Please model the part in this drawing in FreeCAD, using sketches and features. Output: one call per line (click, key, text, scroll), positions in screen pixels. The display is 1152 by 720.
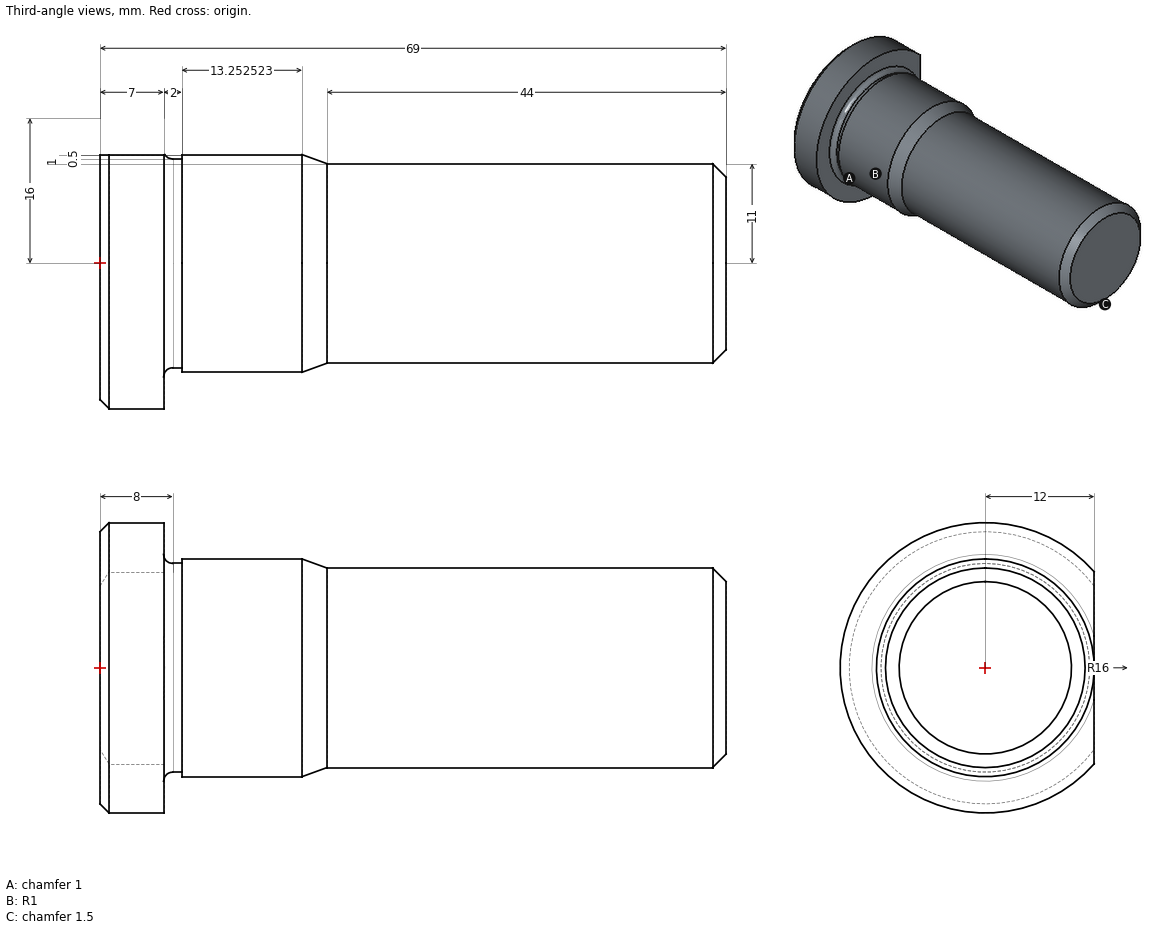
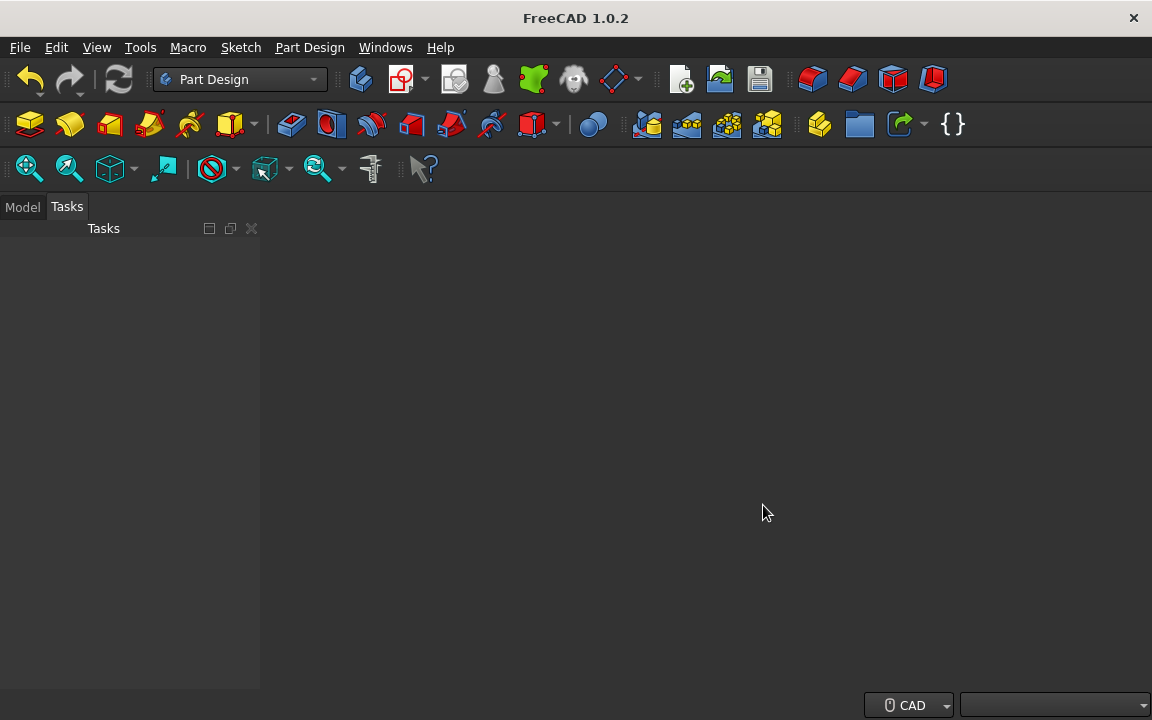
click(680, 80)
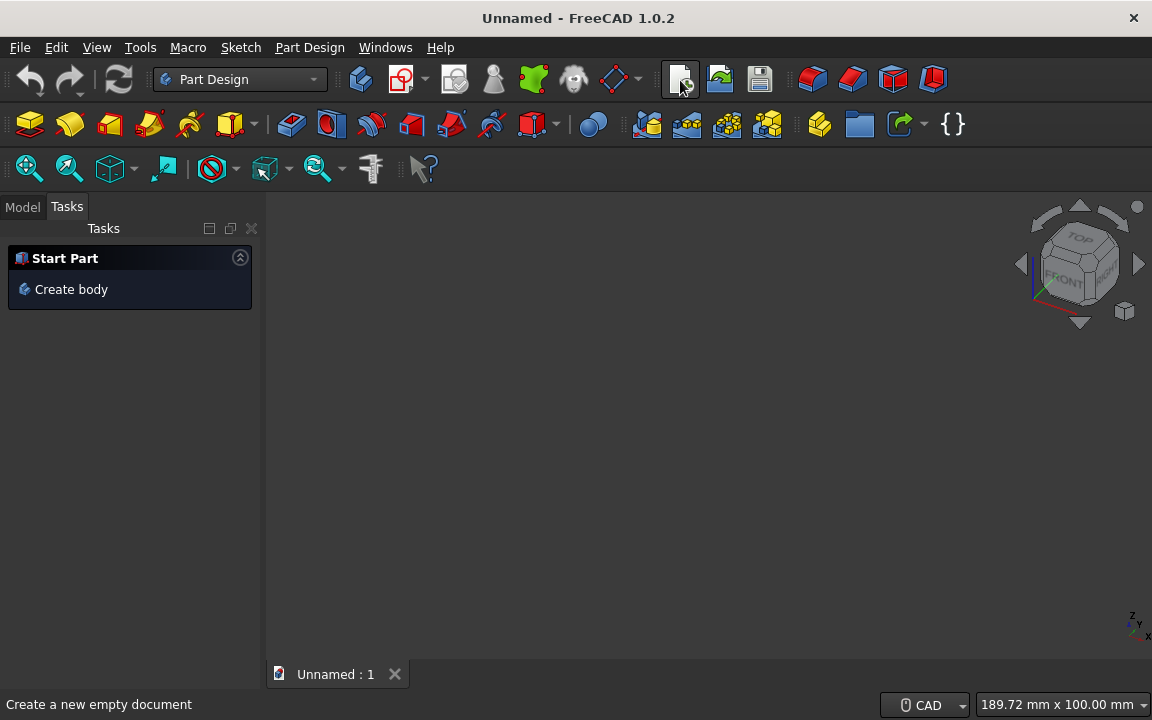
click(402, 80)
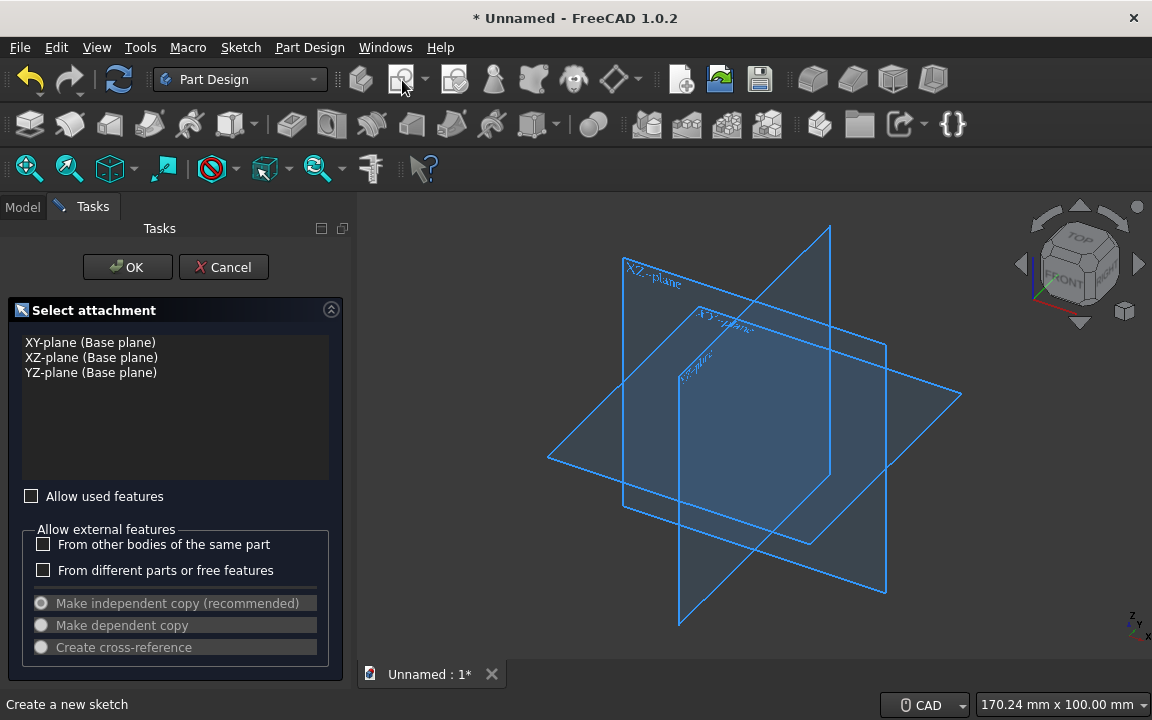
click(82, 342)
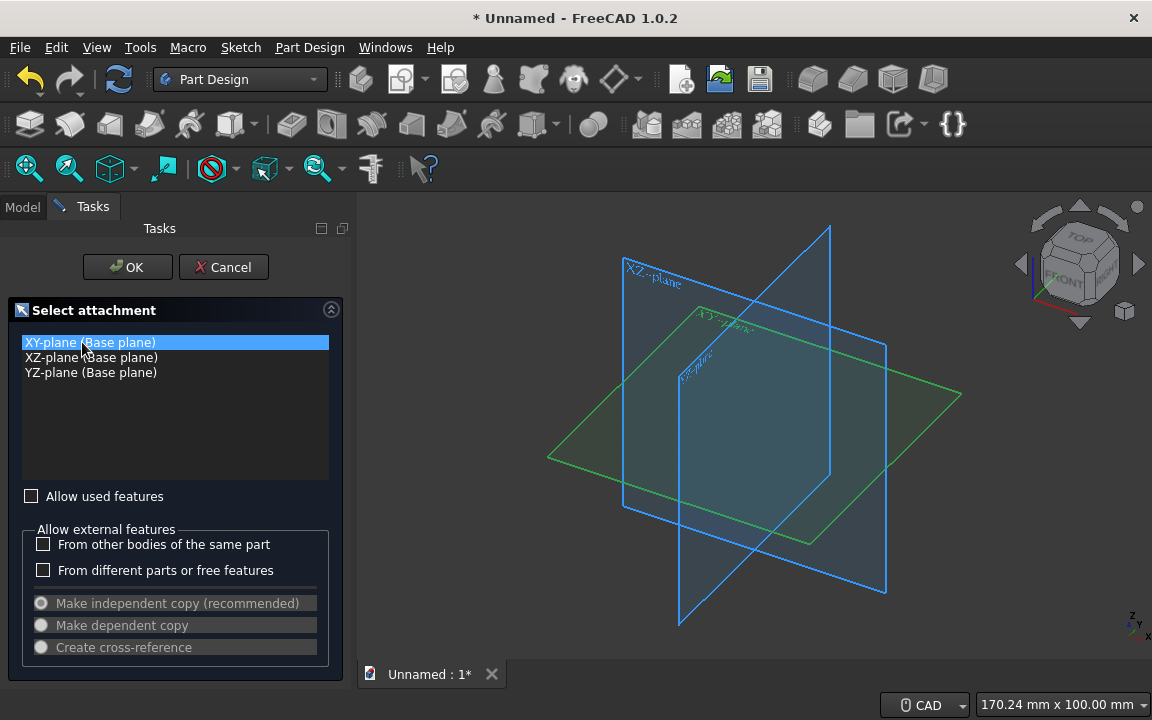
click(128, 267)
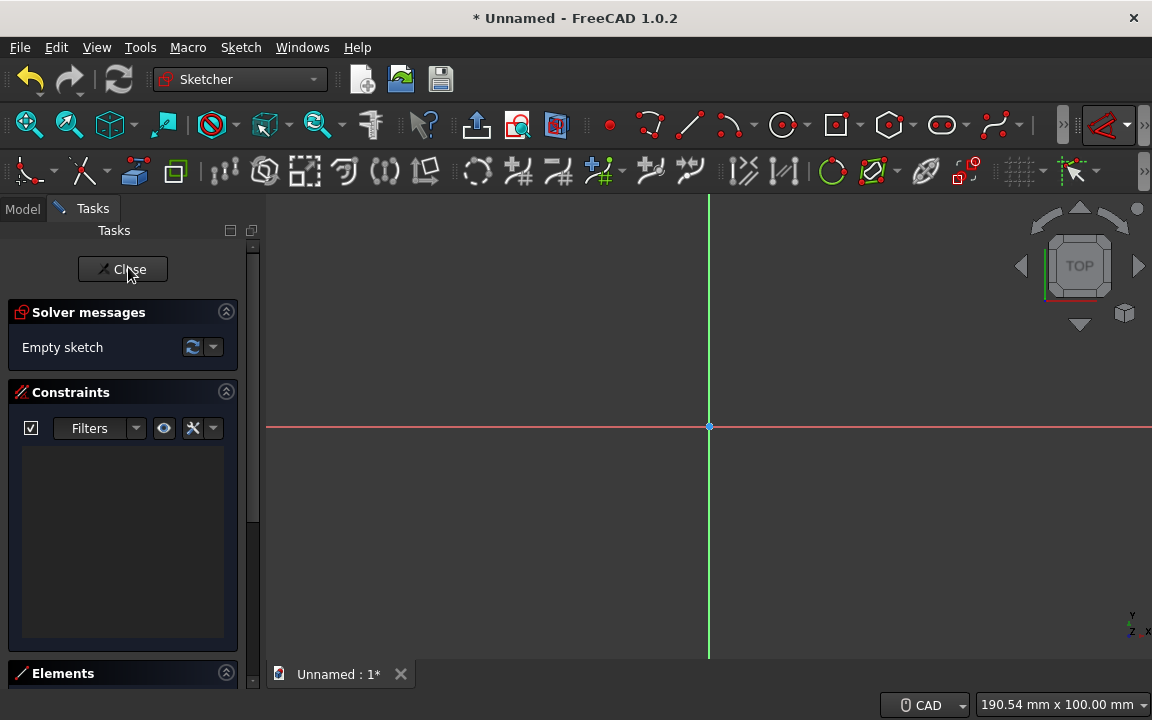
scroll(294, 595, down, 1)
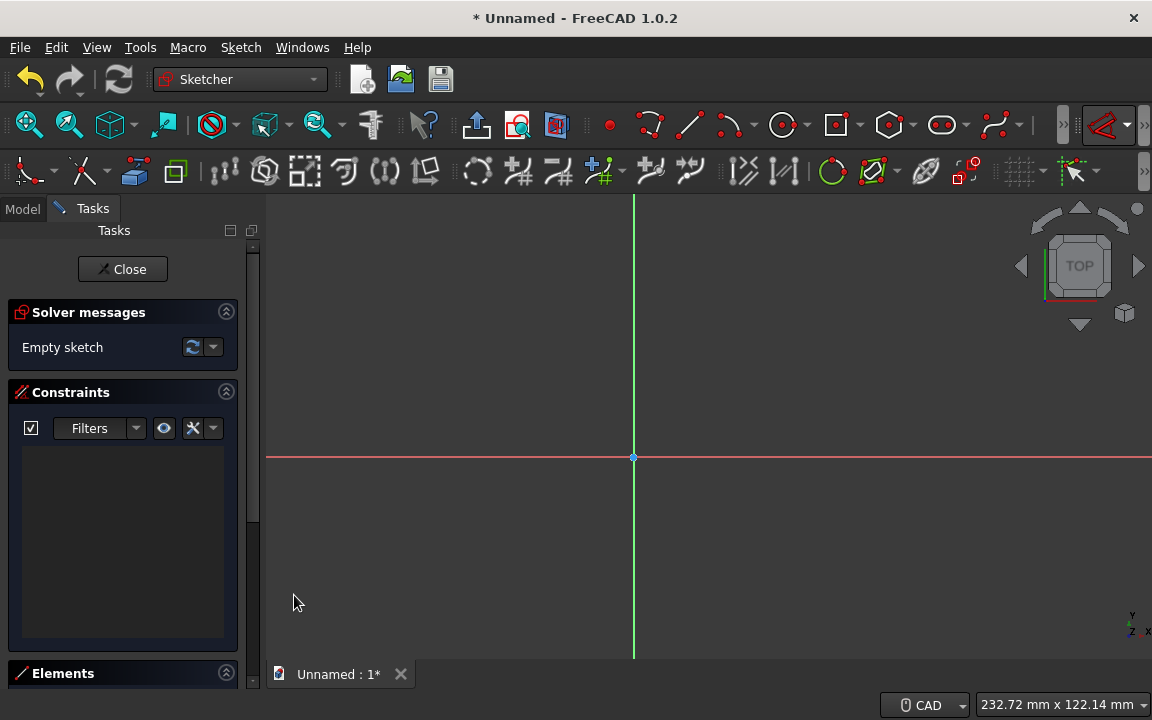
scroll(917, 427, up, 3)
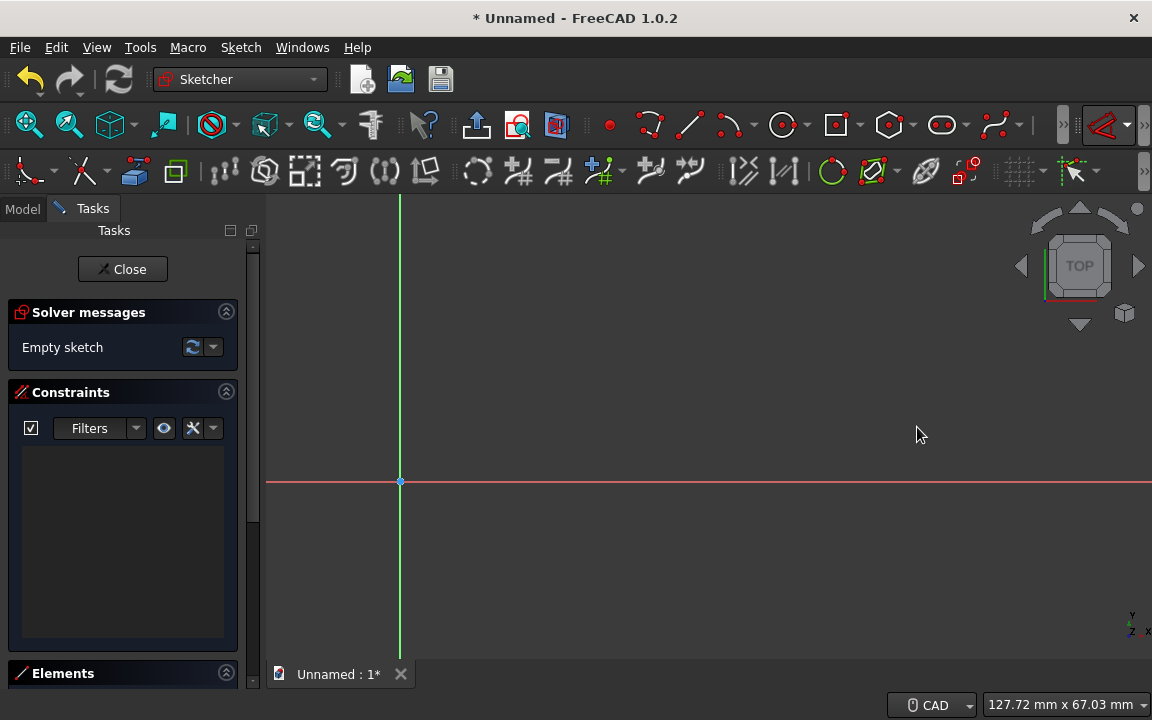
click(650, 126)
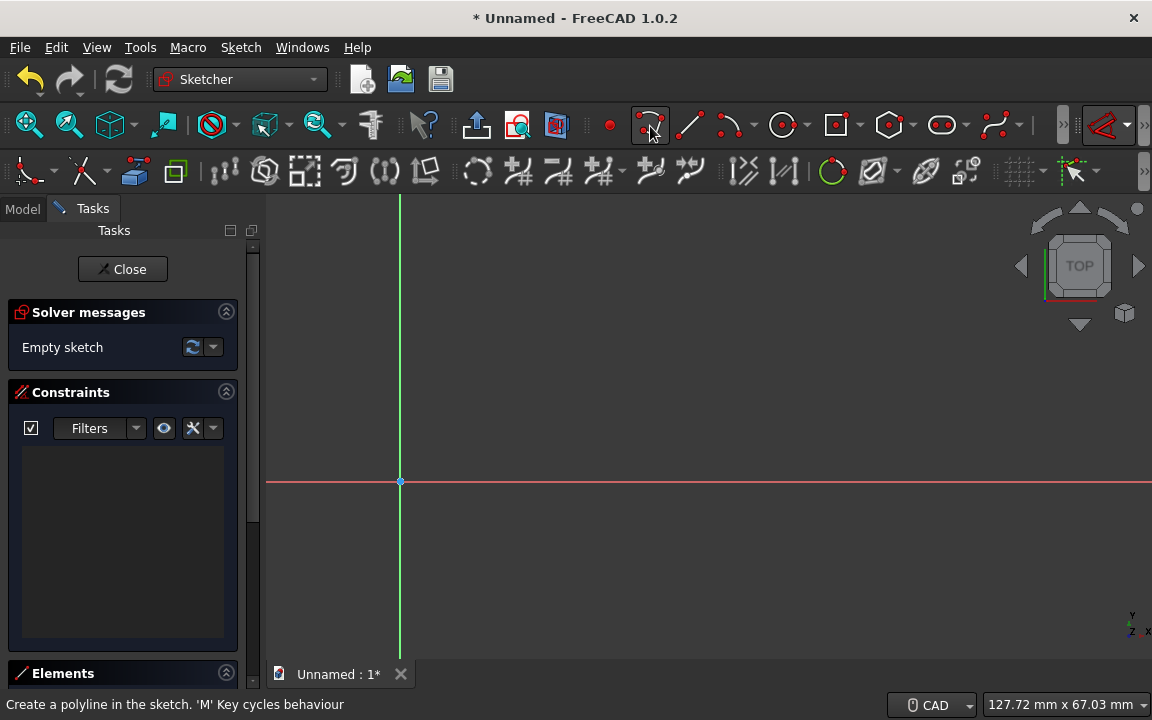
click(400, 482)
click(879, 473)
click(879, 405)
click(574, 405)
click(555, 398)
click(463, 398)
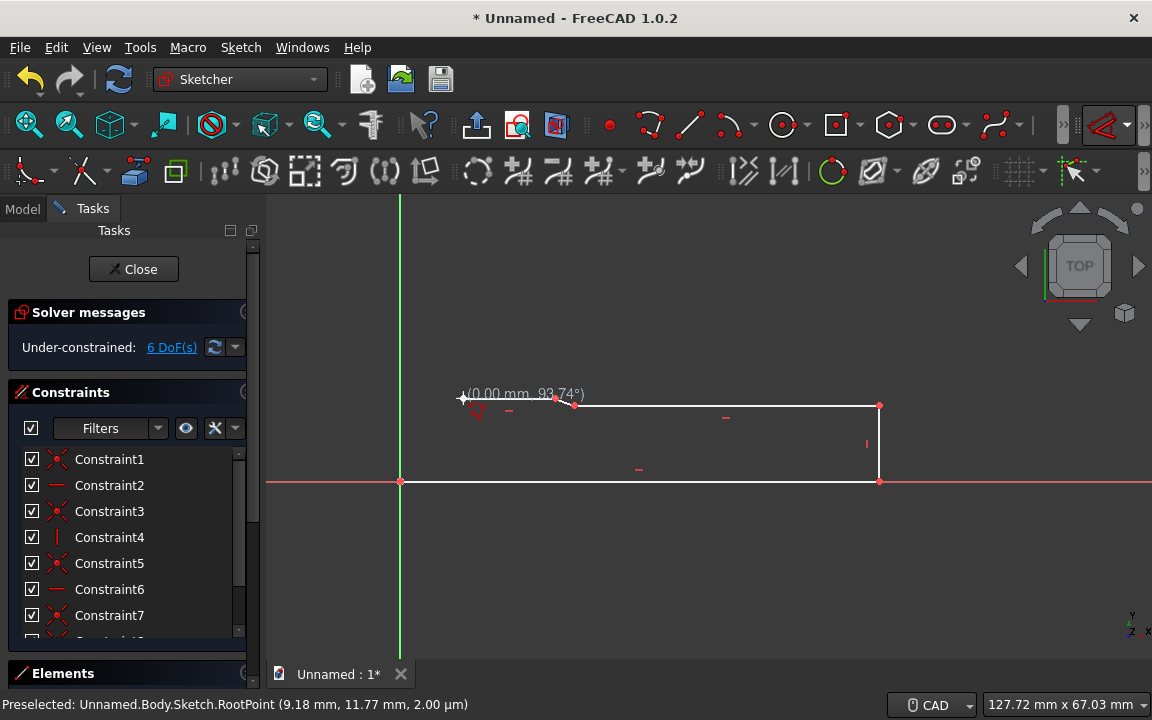
scroll(463, 402, up, 8)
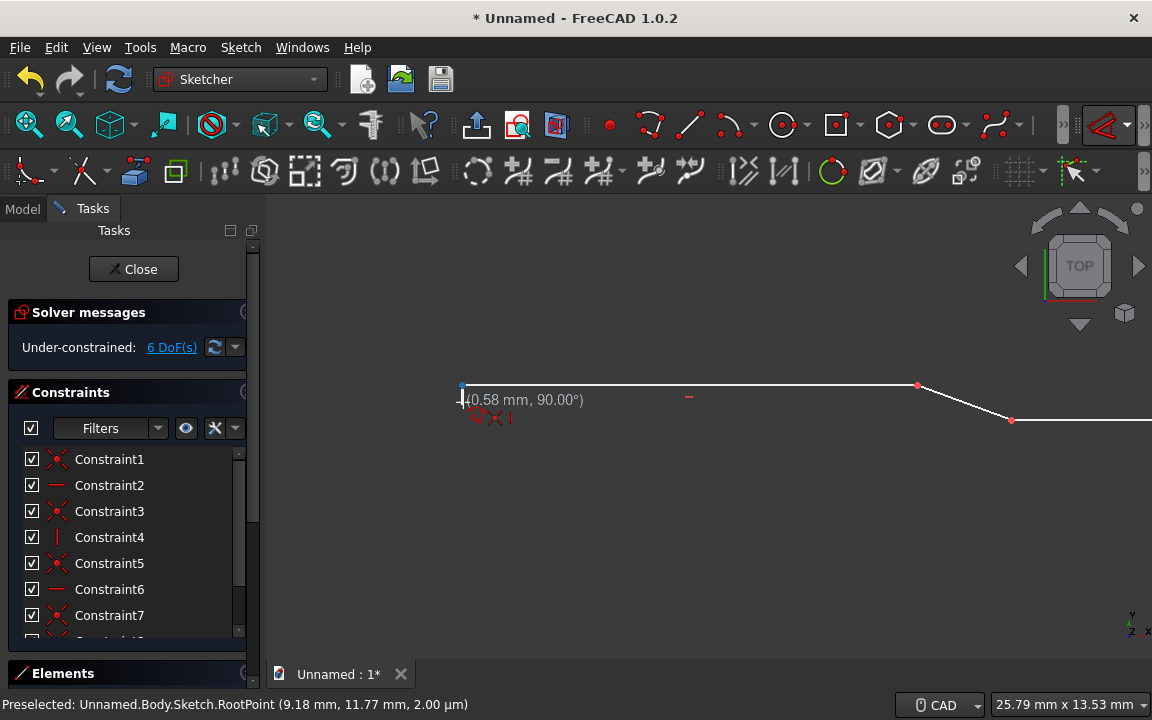
click(462, 399)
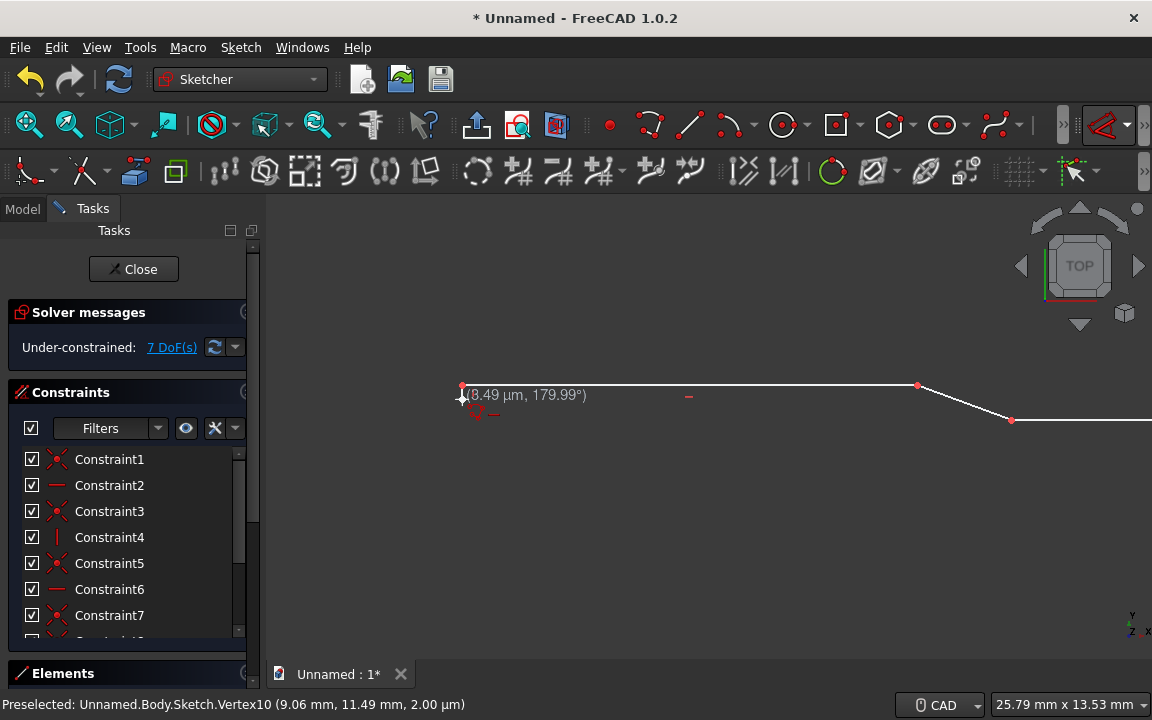
scroll(464, 403, down, 8)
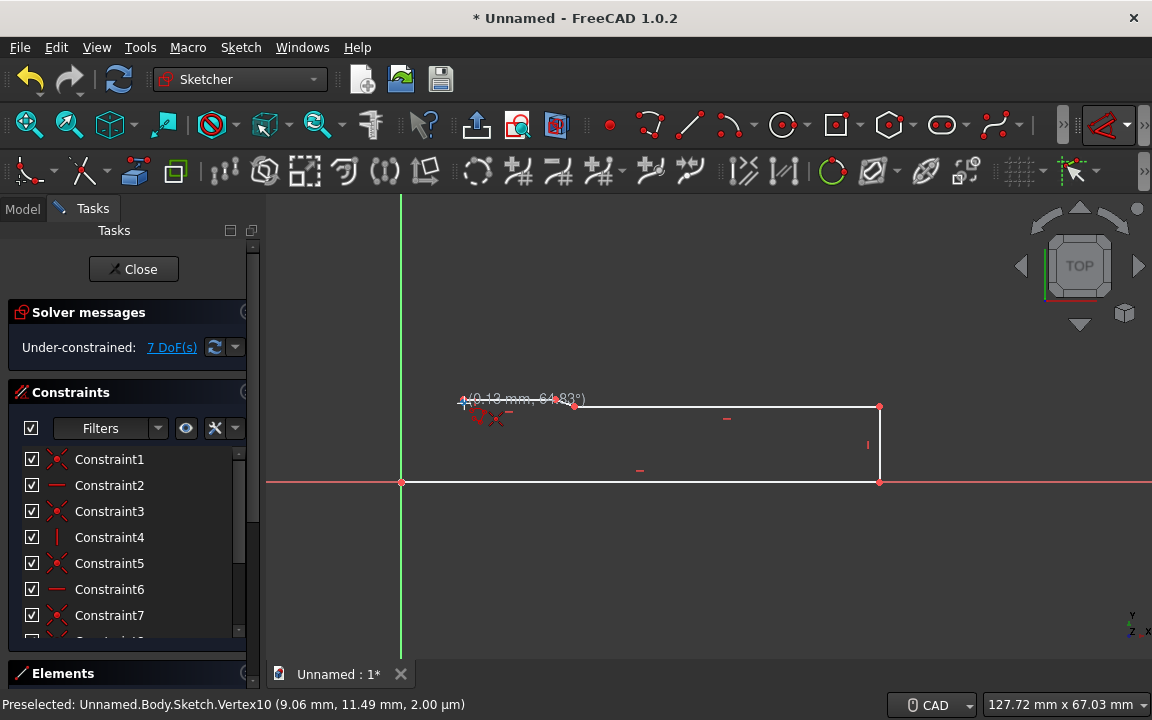
click(450, 403)
click(450, 371)
click(410, 371)
click(401, 482)
key(Escape)
key(Escape)